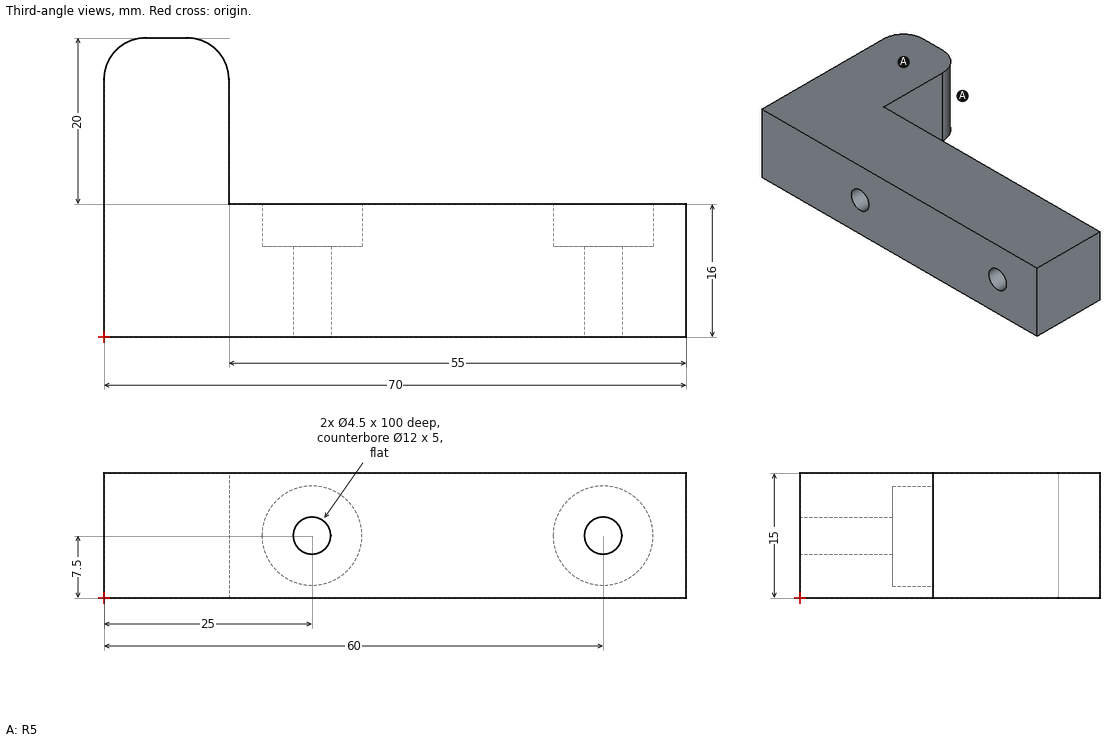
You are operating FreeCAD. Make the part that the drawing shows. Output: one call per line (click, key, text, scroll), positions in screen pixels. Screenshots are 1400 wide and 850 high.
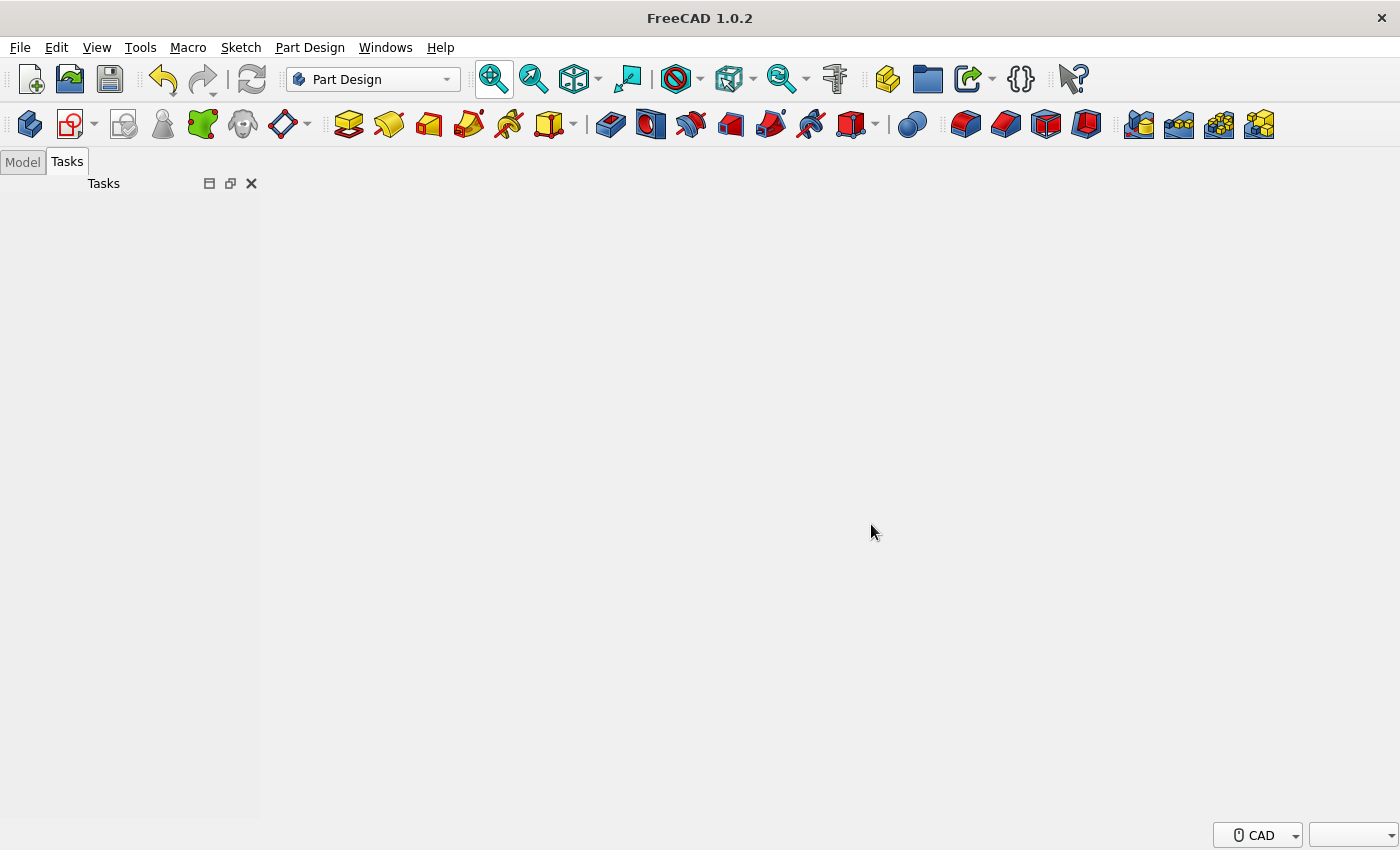
click(30, 80)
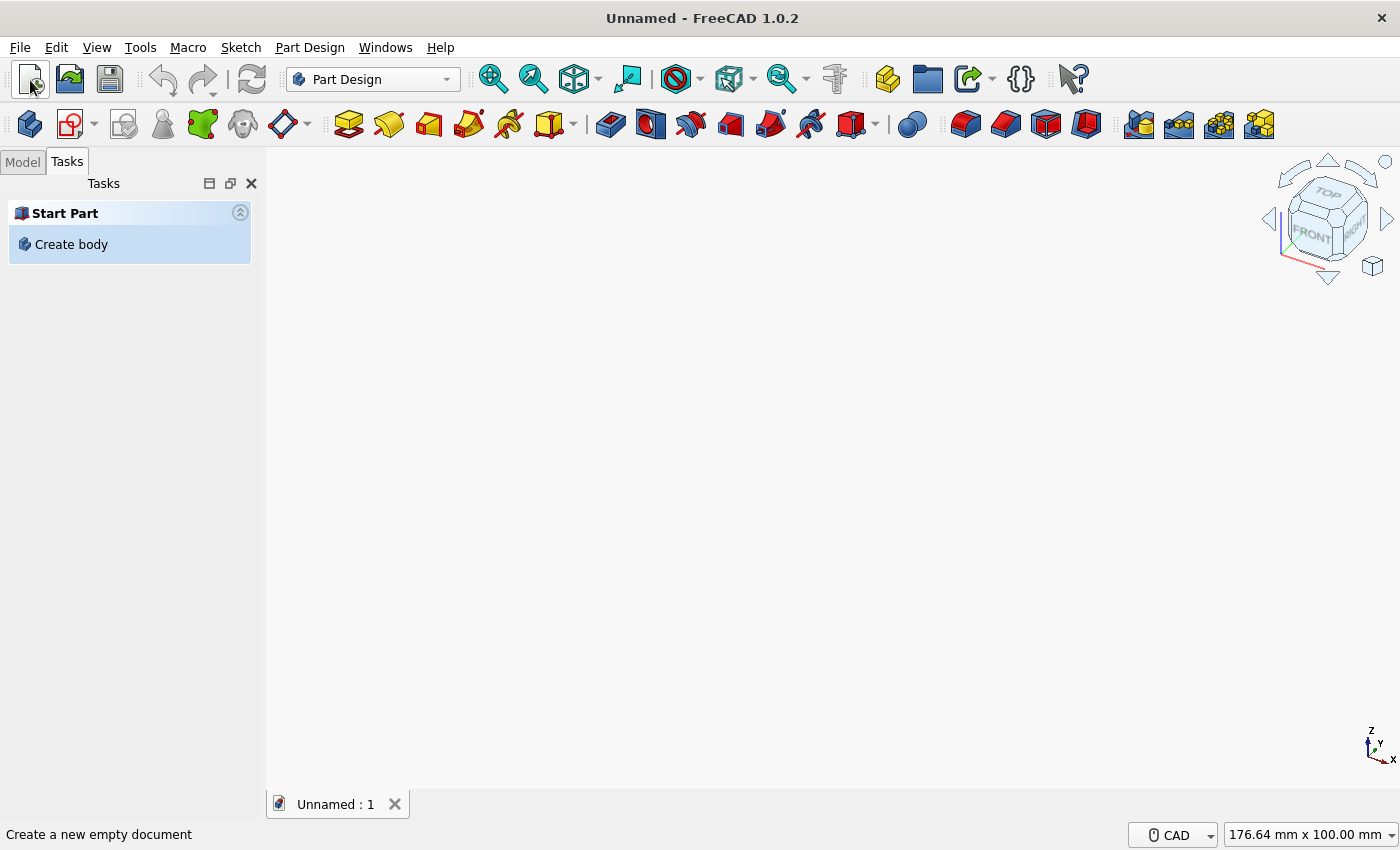
click(70, 124)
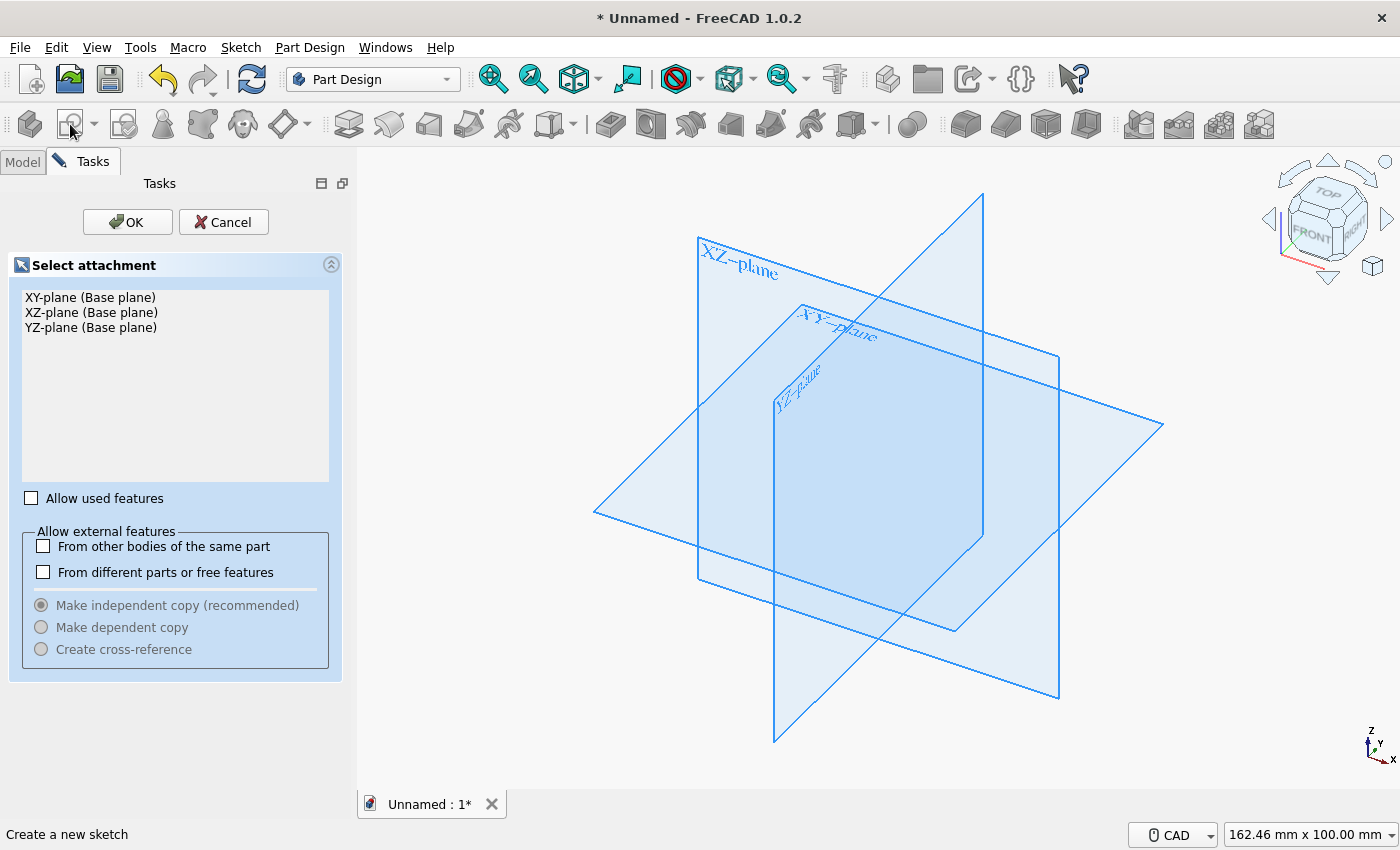
click(82, 298)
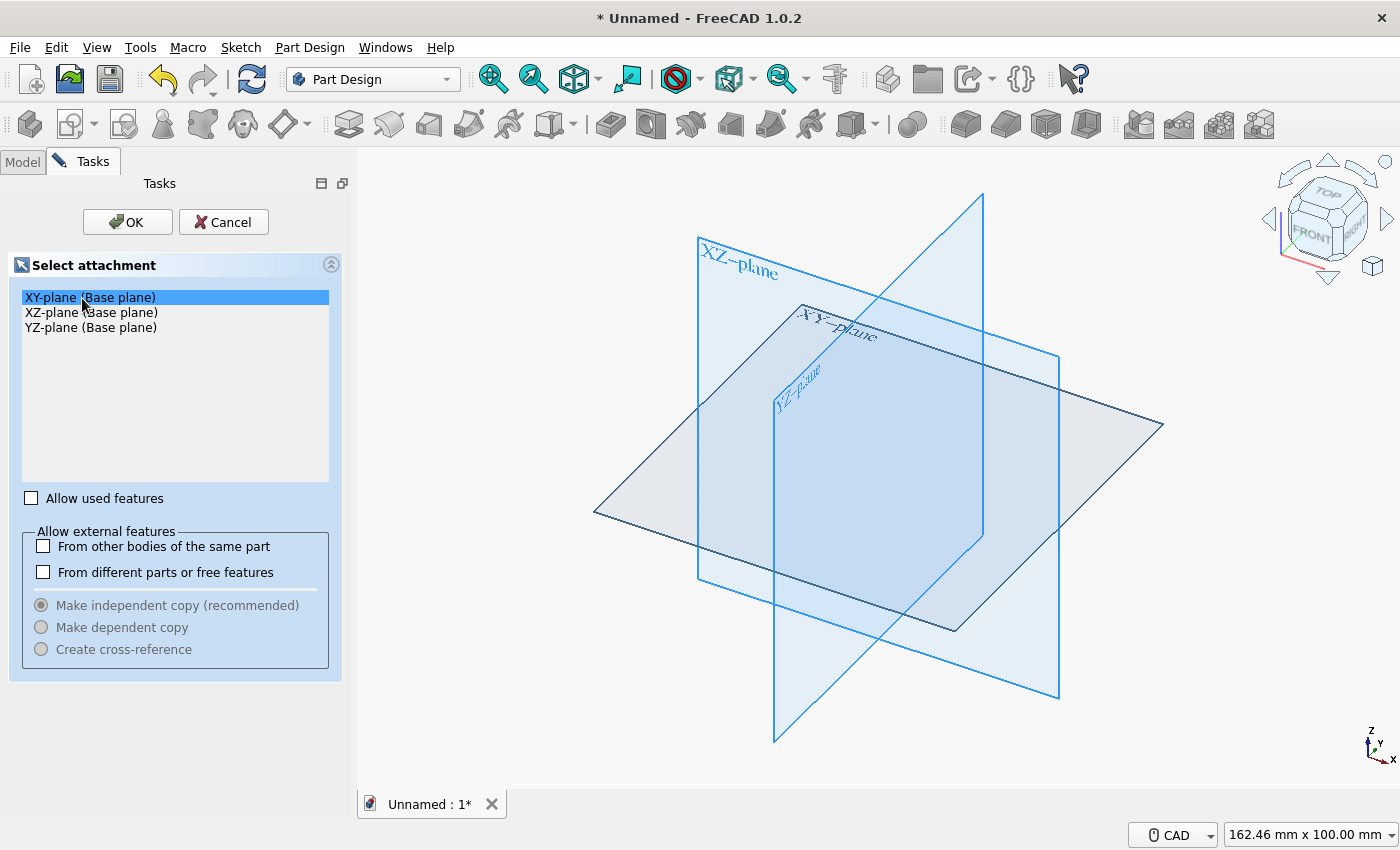
click(128, 222)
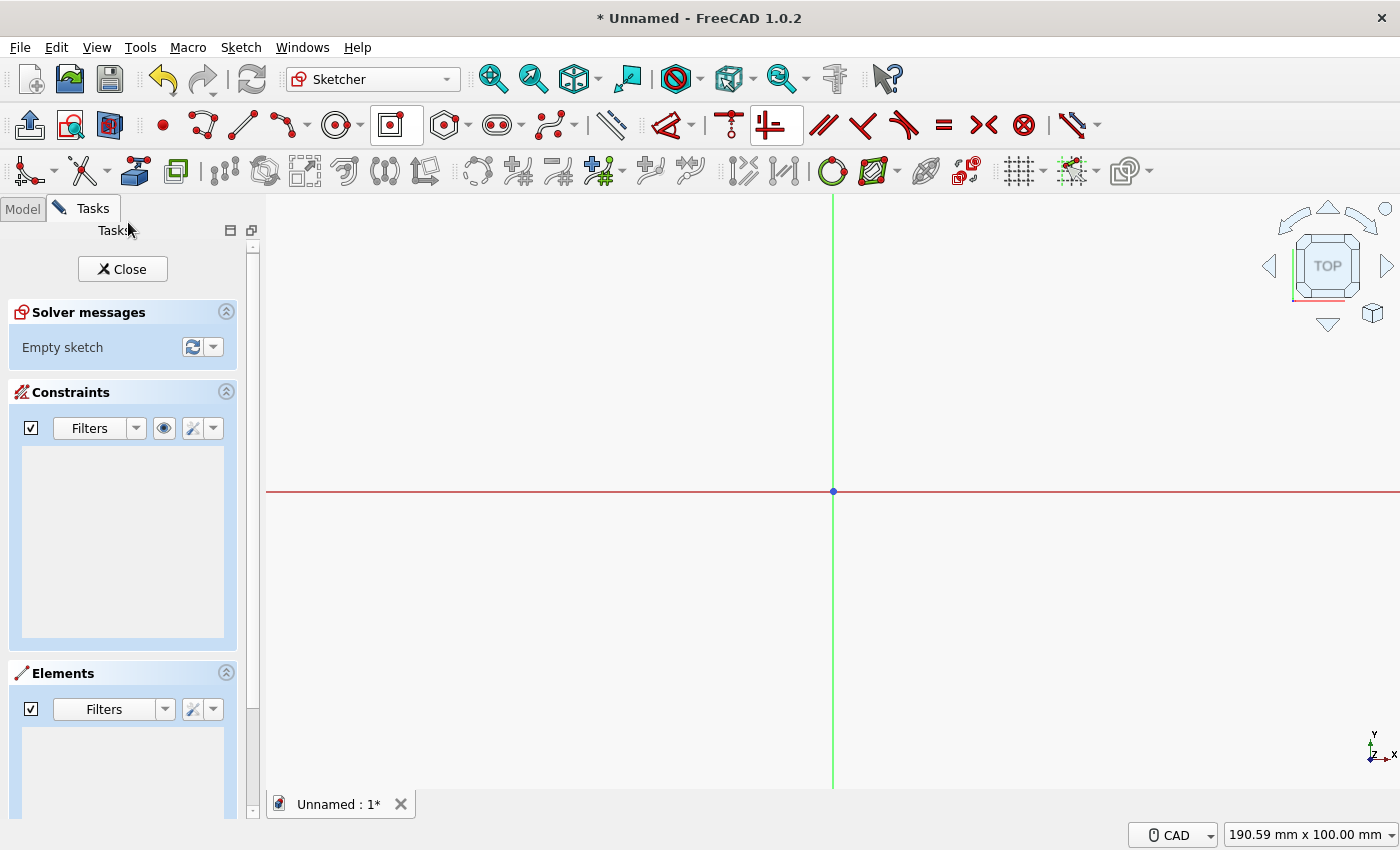
scroll(294, 761, down, 1)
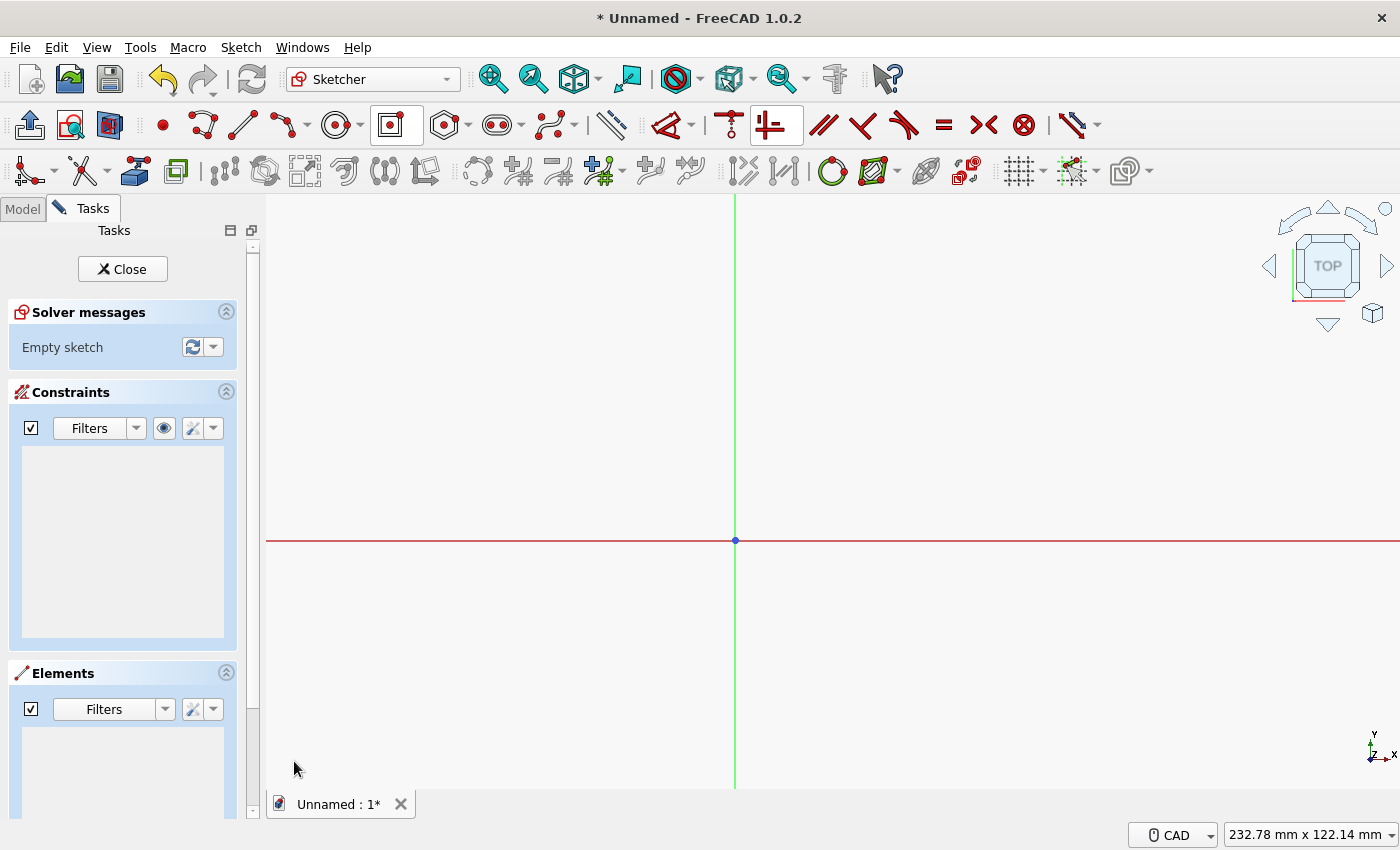
scroll(1078, 406, up, 3)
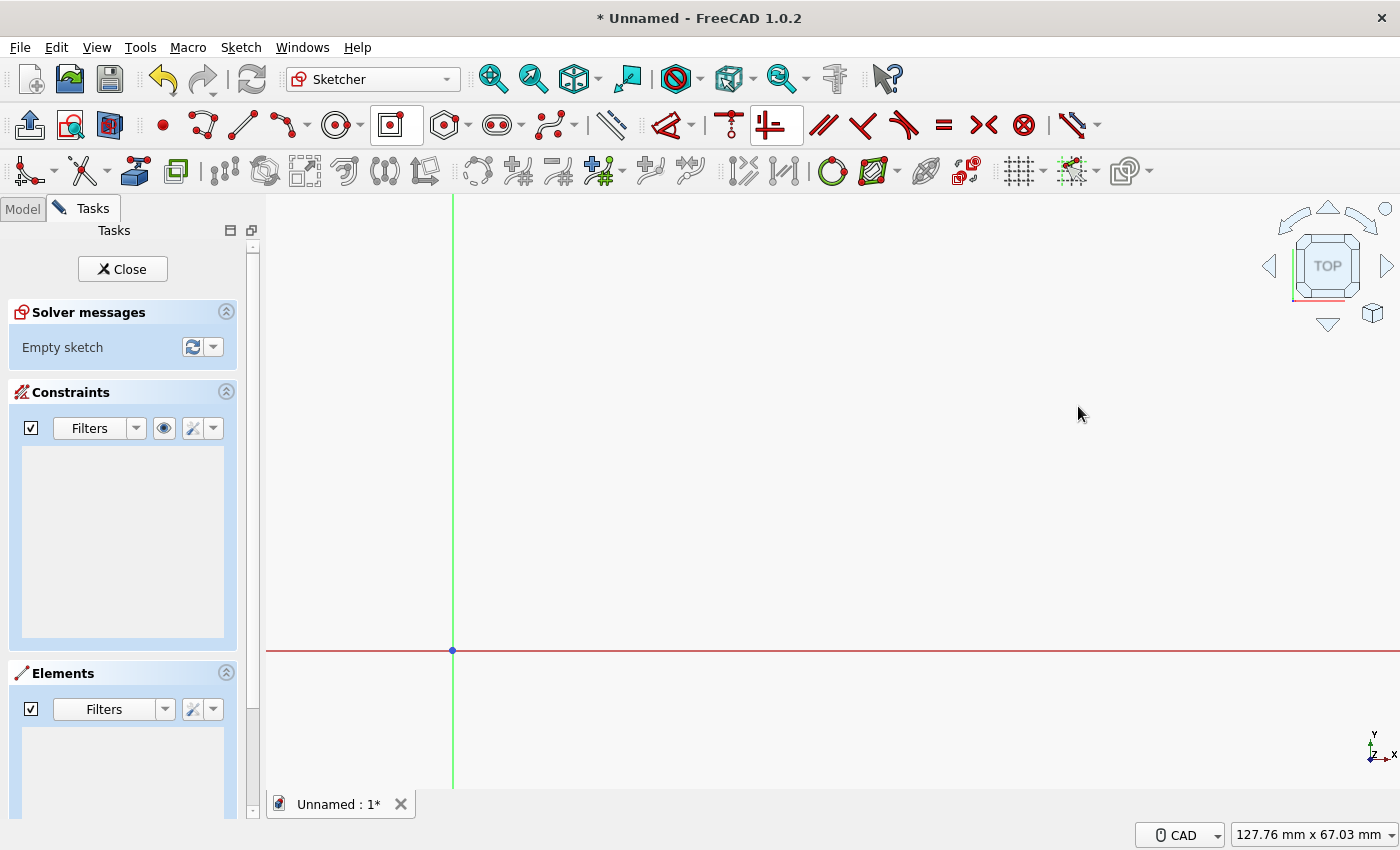
click(204, 126)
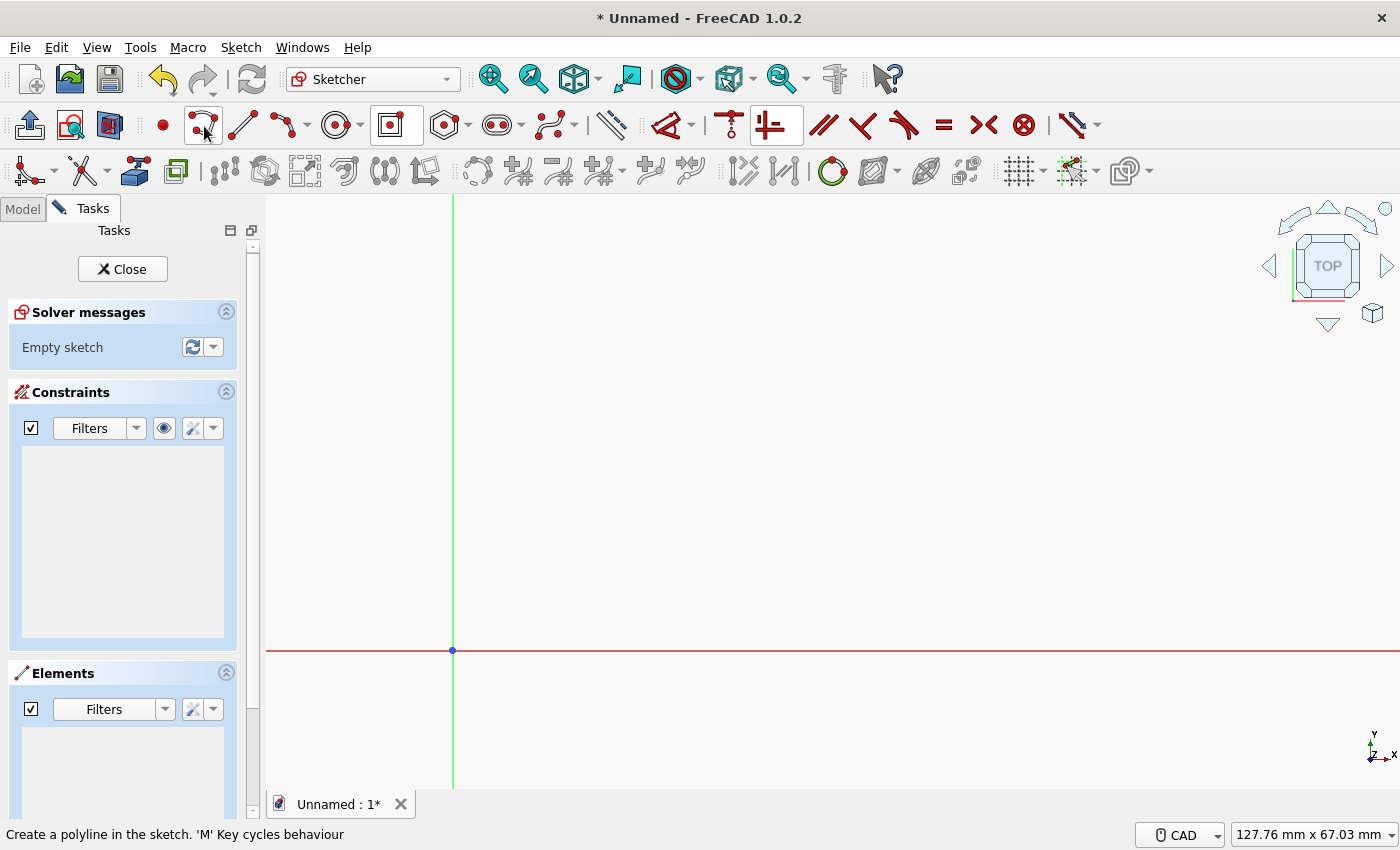
click(453, 651)
click(1074, 642)
click(1074, 509)
click(586, 509)
click(586, 331)
click(462, 331)
click(453, 651)
key(Escape)
key(Escape)